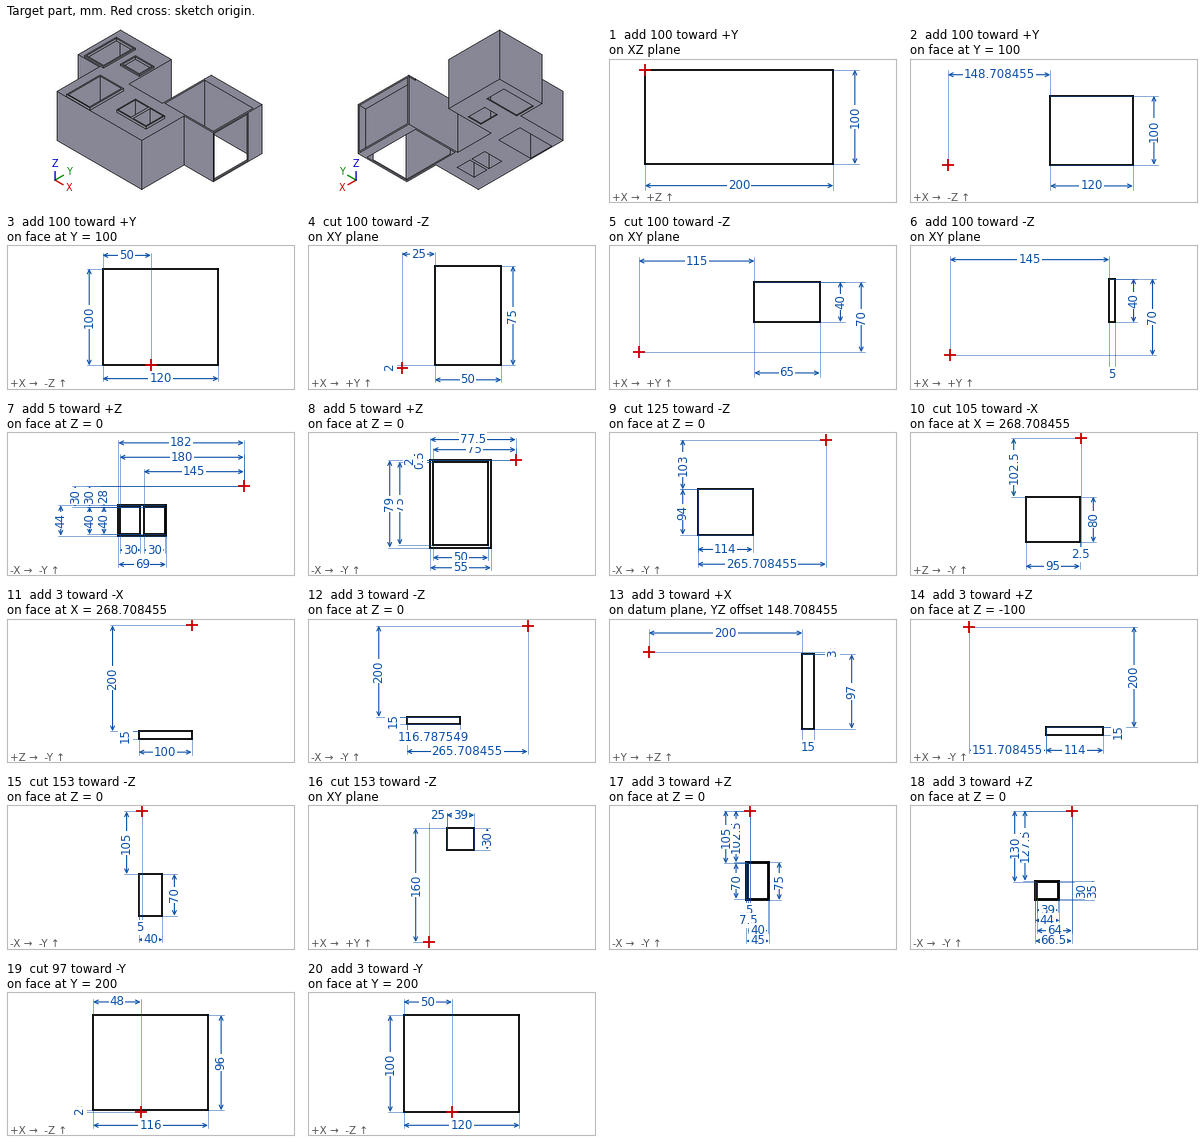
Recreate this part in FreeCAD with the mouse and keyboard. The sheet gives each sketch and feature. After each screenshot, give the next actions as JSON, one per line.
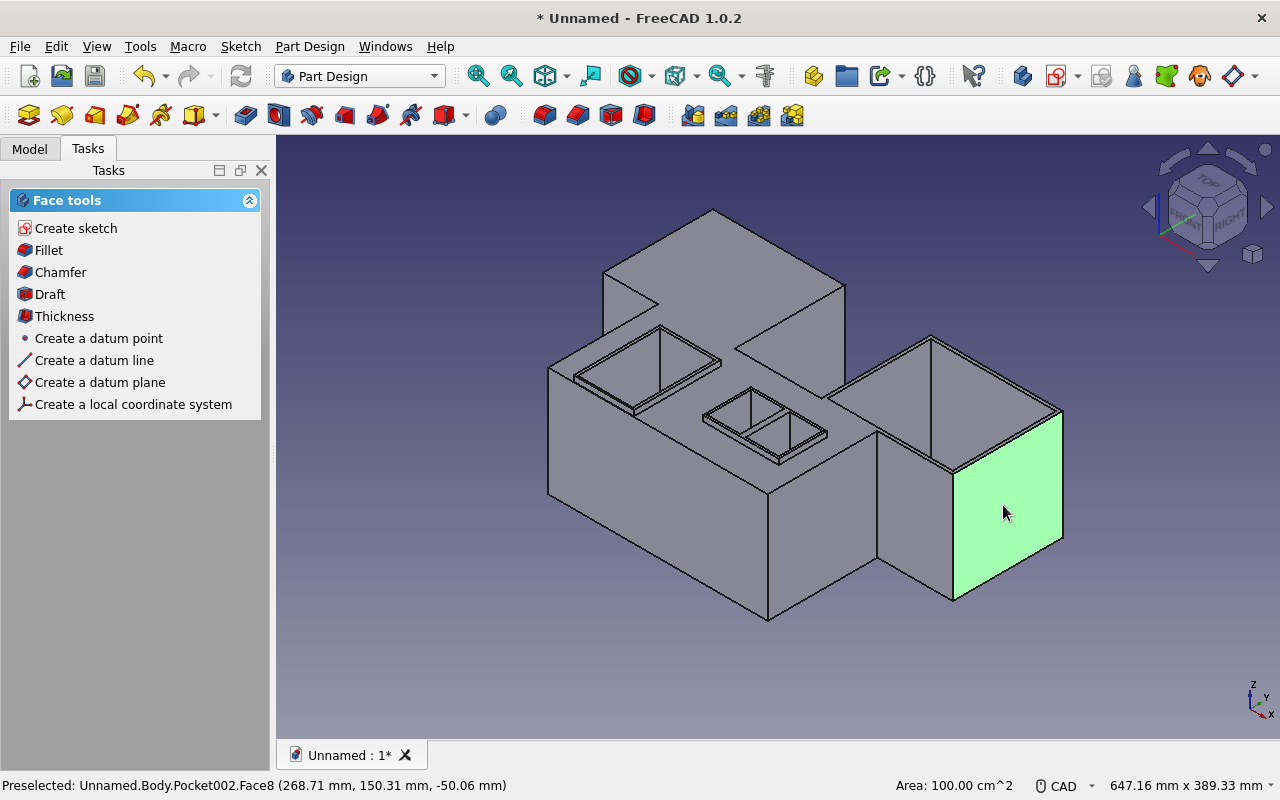
{"action": "left_click", "coordinate": [1056, 76]}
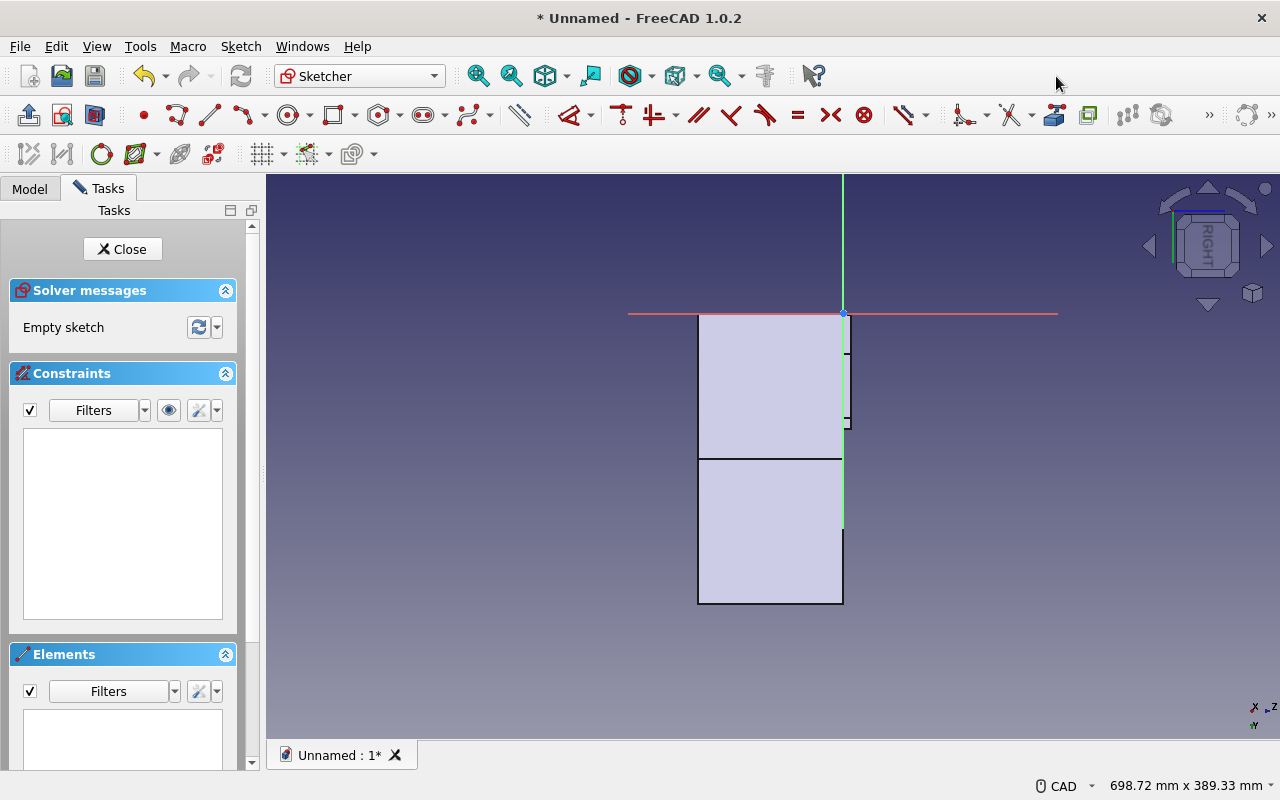
{"action": "scroll", "coordinate": [911, 425], "scroll_direction": "up", "scroll_amount": 2}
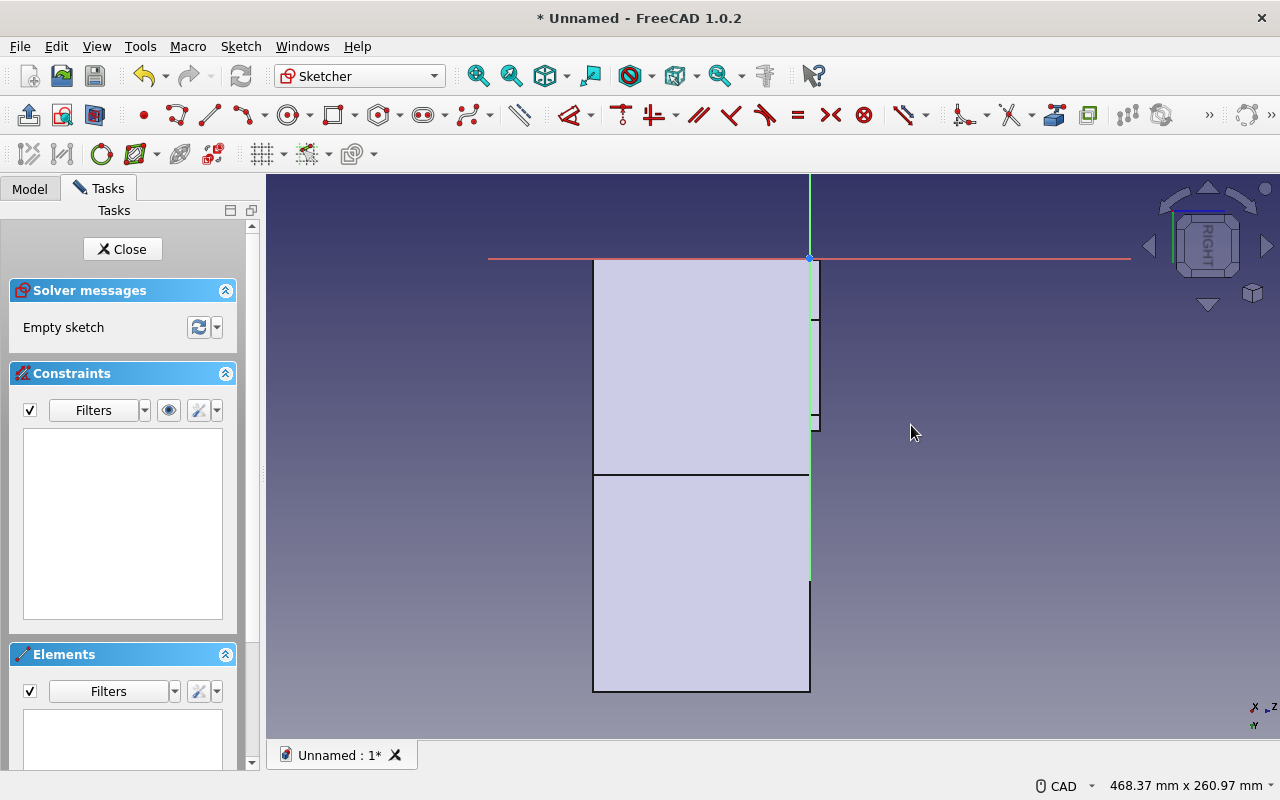
{"action": "left_click", "coordinate": [332, 116]}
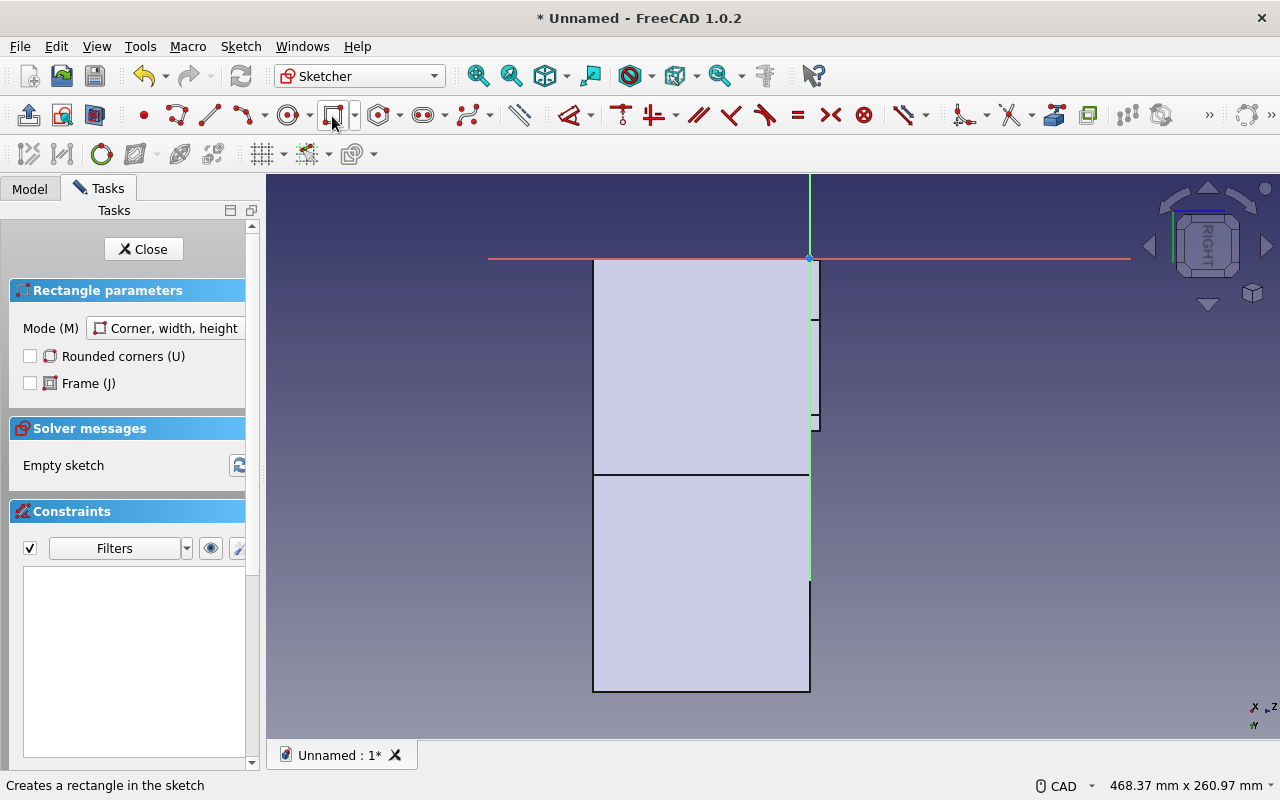
{"action": "left_click", "coordinate": [599, 481]}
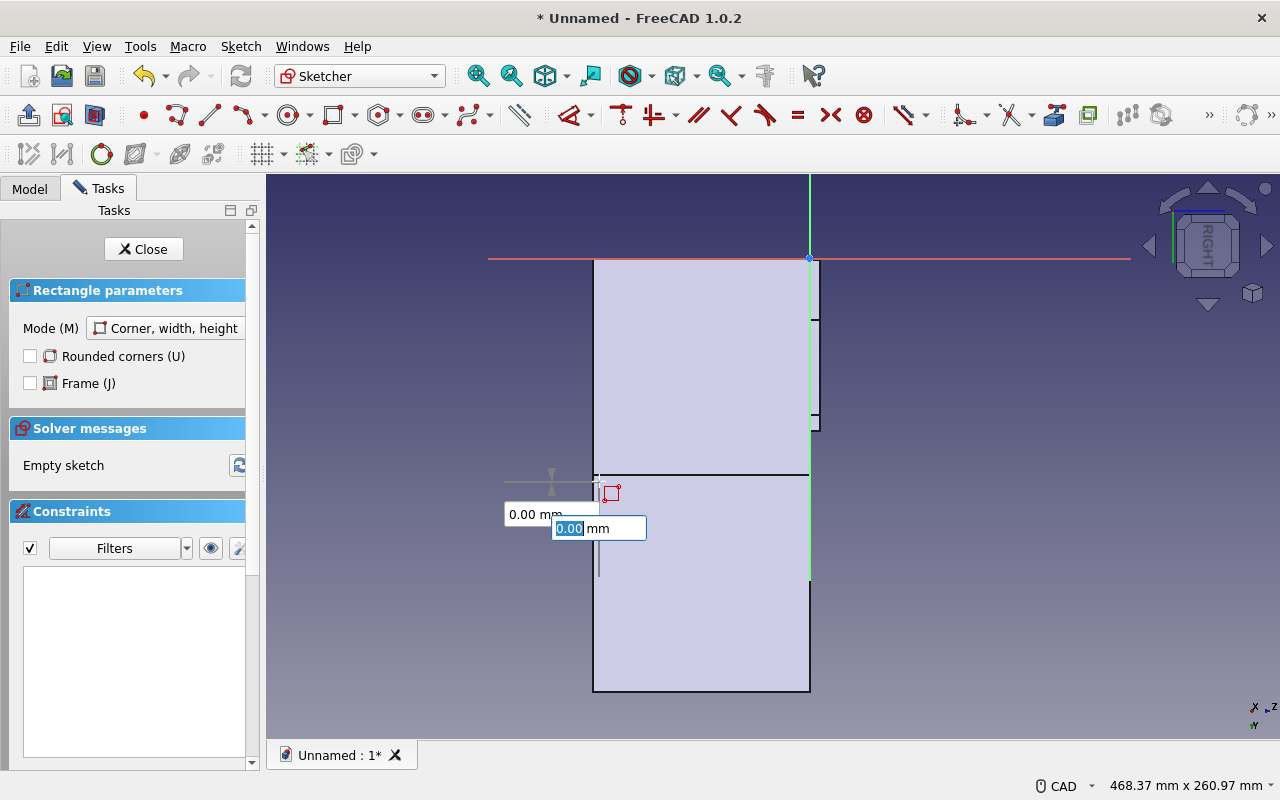
{"action": "scroll", "coordinate": [804, 654], "scroll_direction": "up", "scroll_amount": 6}
{"action": "mouse_move", "coordinate": [804, 652]}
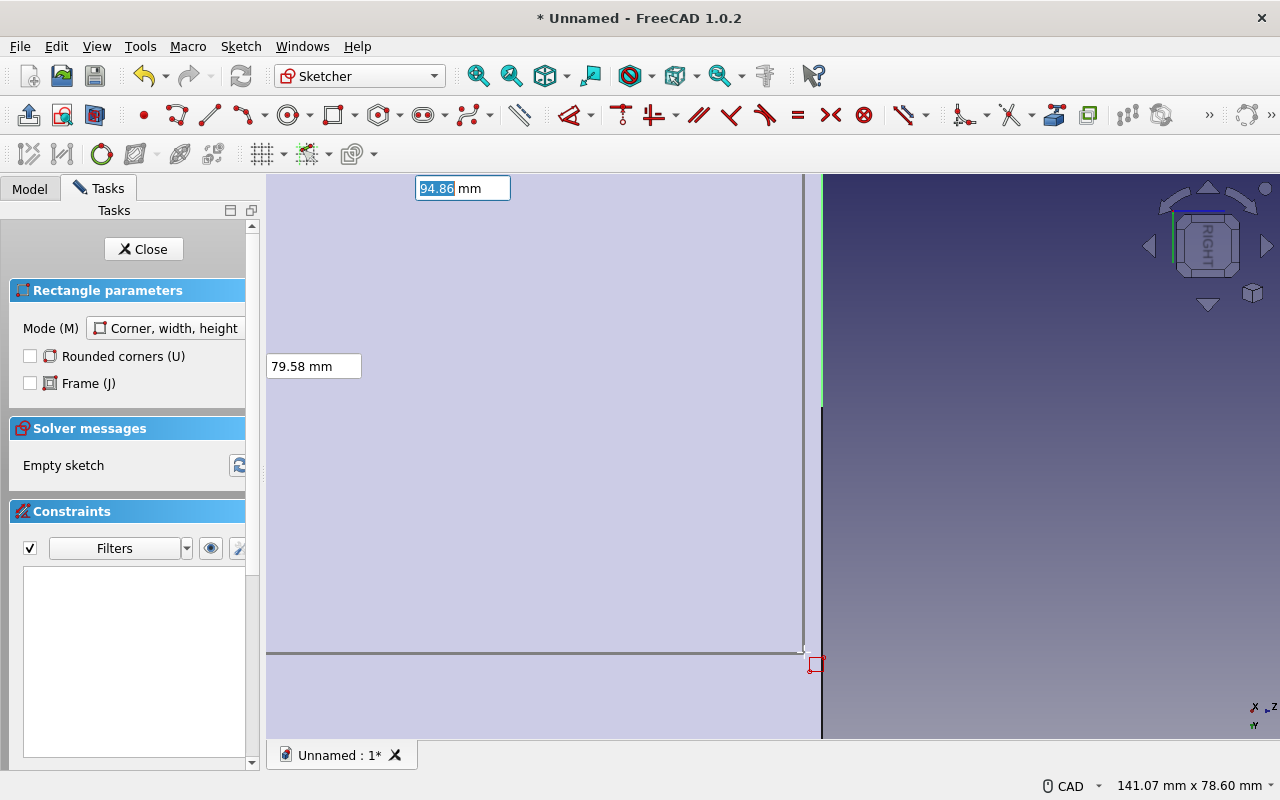
{"action": "type", "text": "95"}
{"action": "key", "text": "Tab"}
{"action": "type", "text": "80"}
{"action": "key", "text": "Return"}
{"action": "key", "text": "Escape"}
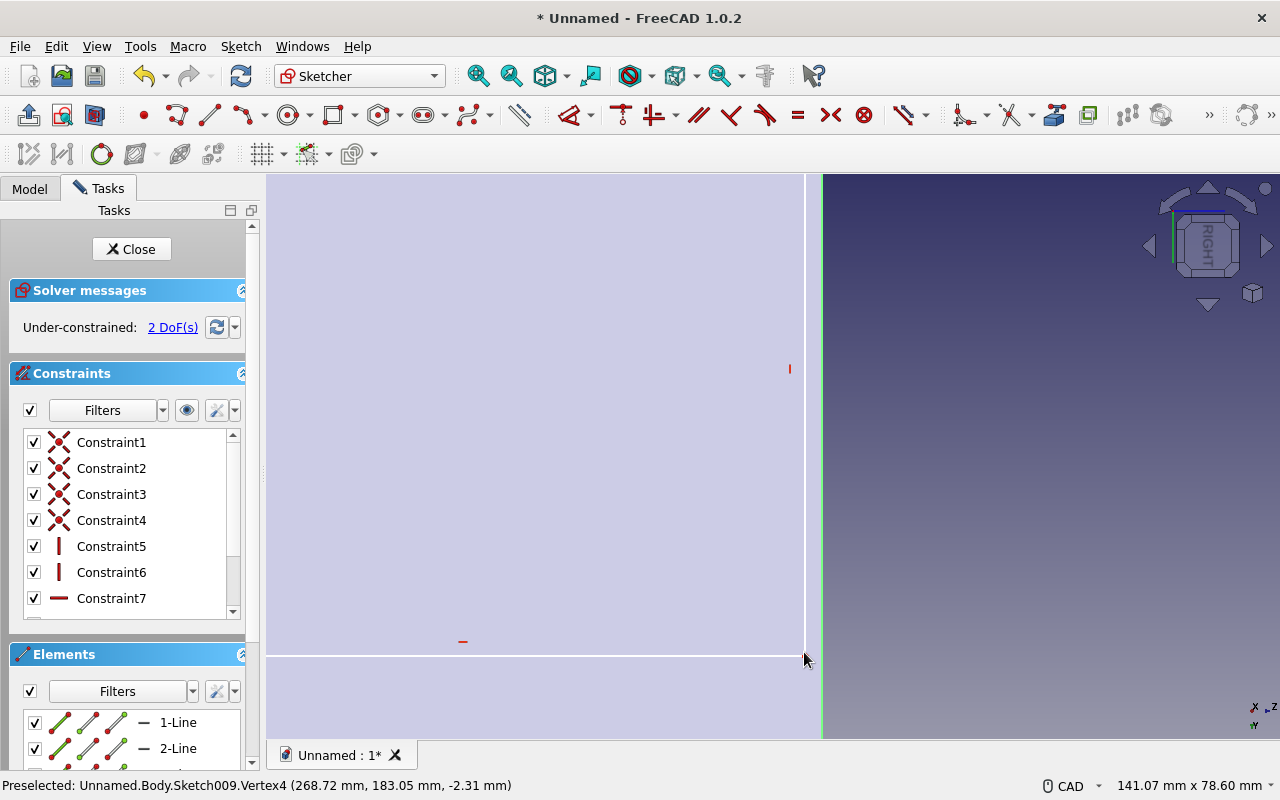
{"action": "left_click", "coordinate": [568, 116]}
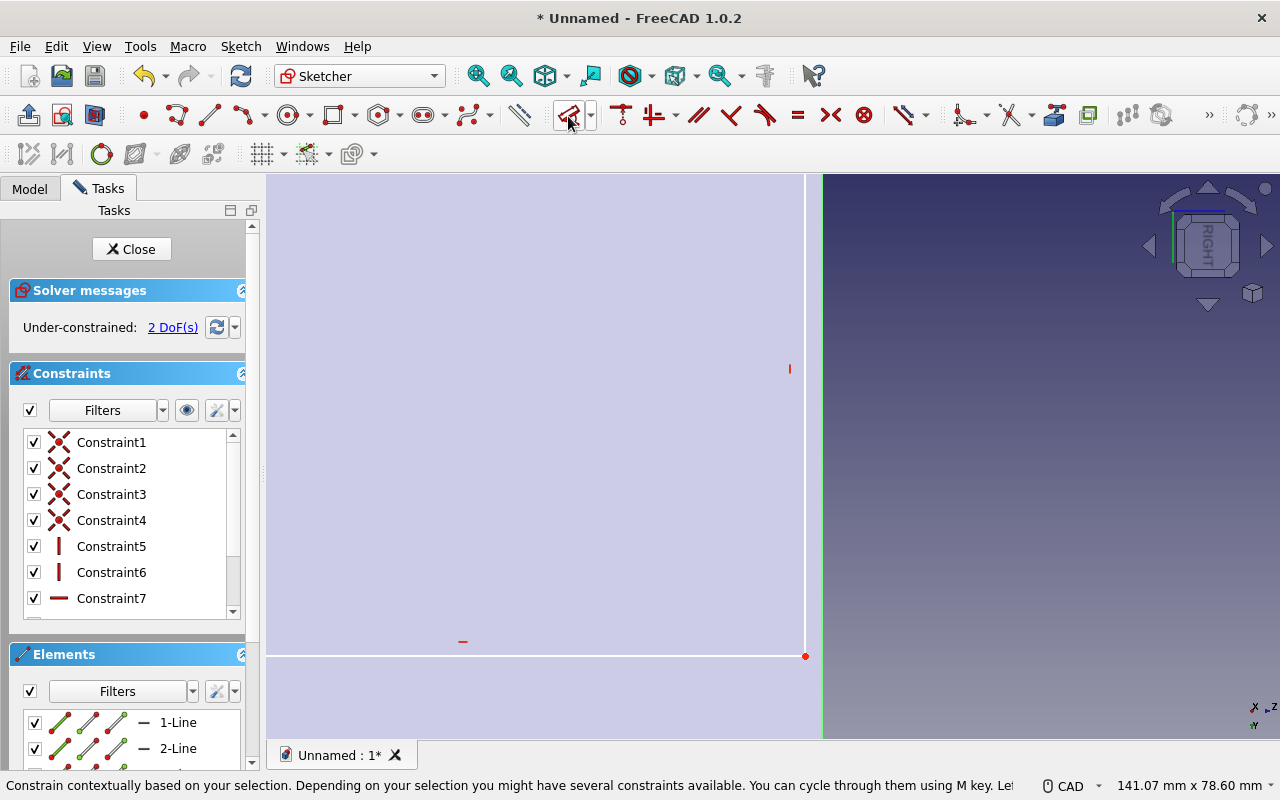
{"action": "scroll", "coordinate": [805, 656], "scroll_direction": "up", "scroll_amount": 4}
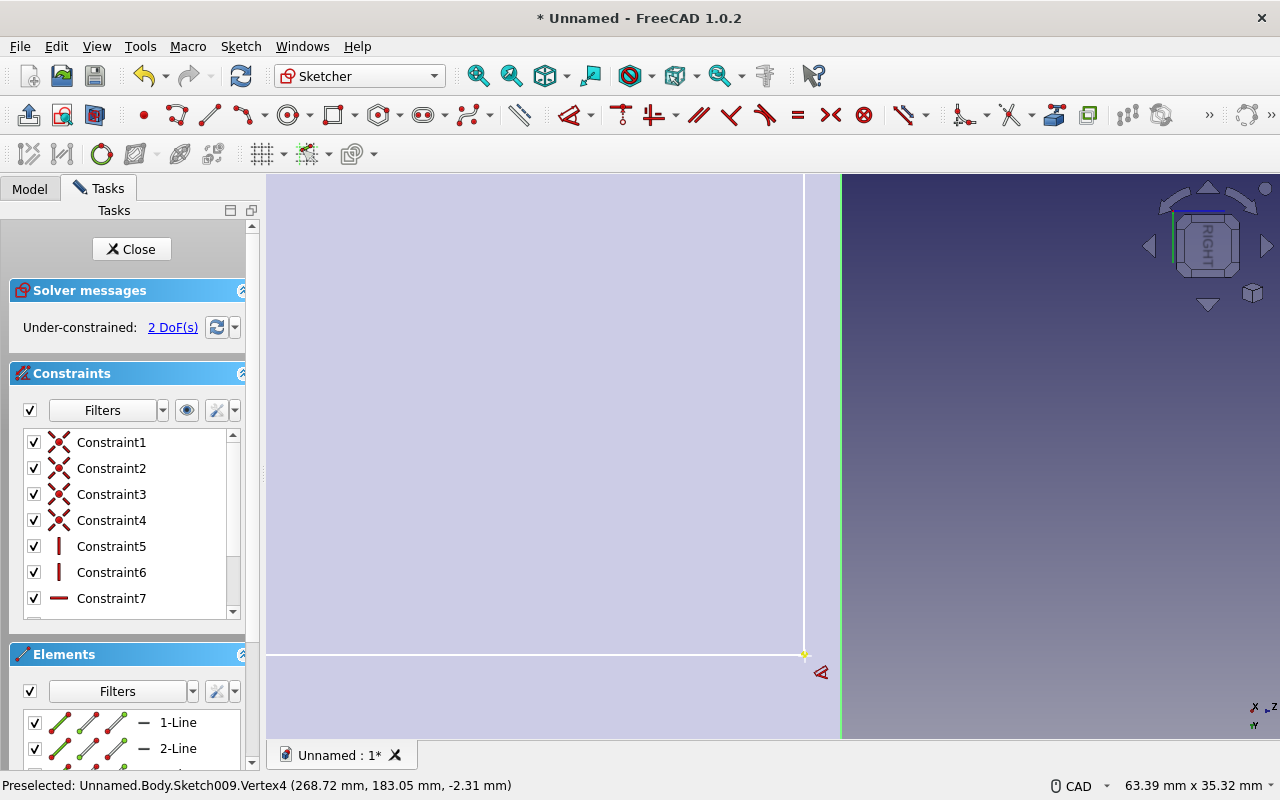
{"action": "left_click", "coordinate": [804, 655]}
{"action": "left_click", "coordinate": [823, 689]}